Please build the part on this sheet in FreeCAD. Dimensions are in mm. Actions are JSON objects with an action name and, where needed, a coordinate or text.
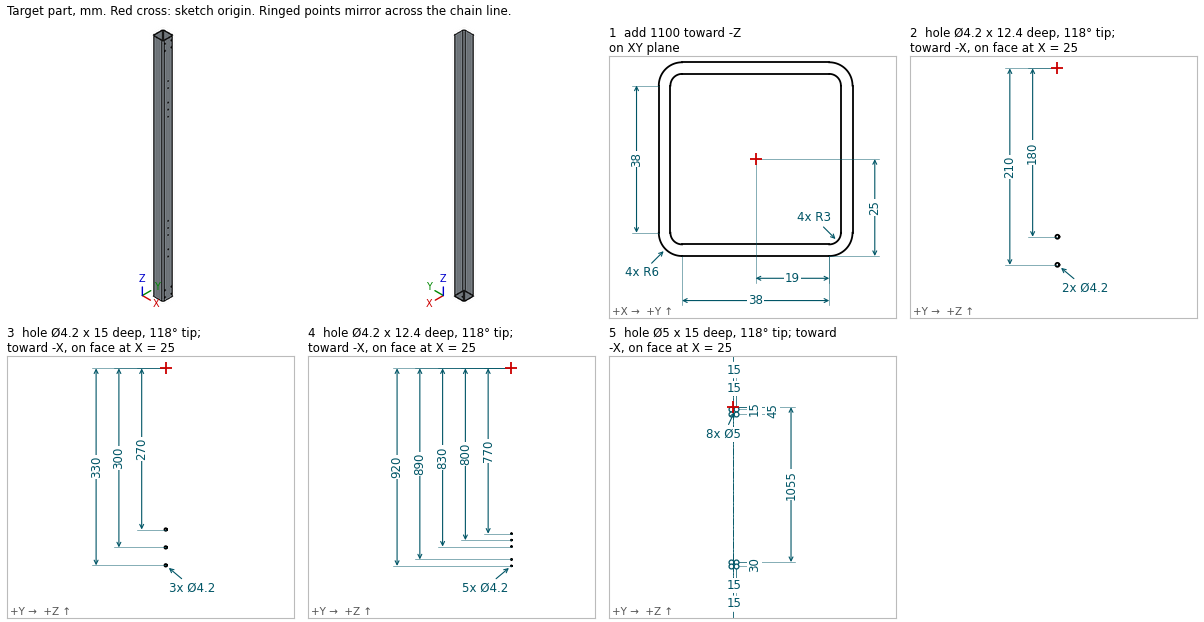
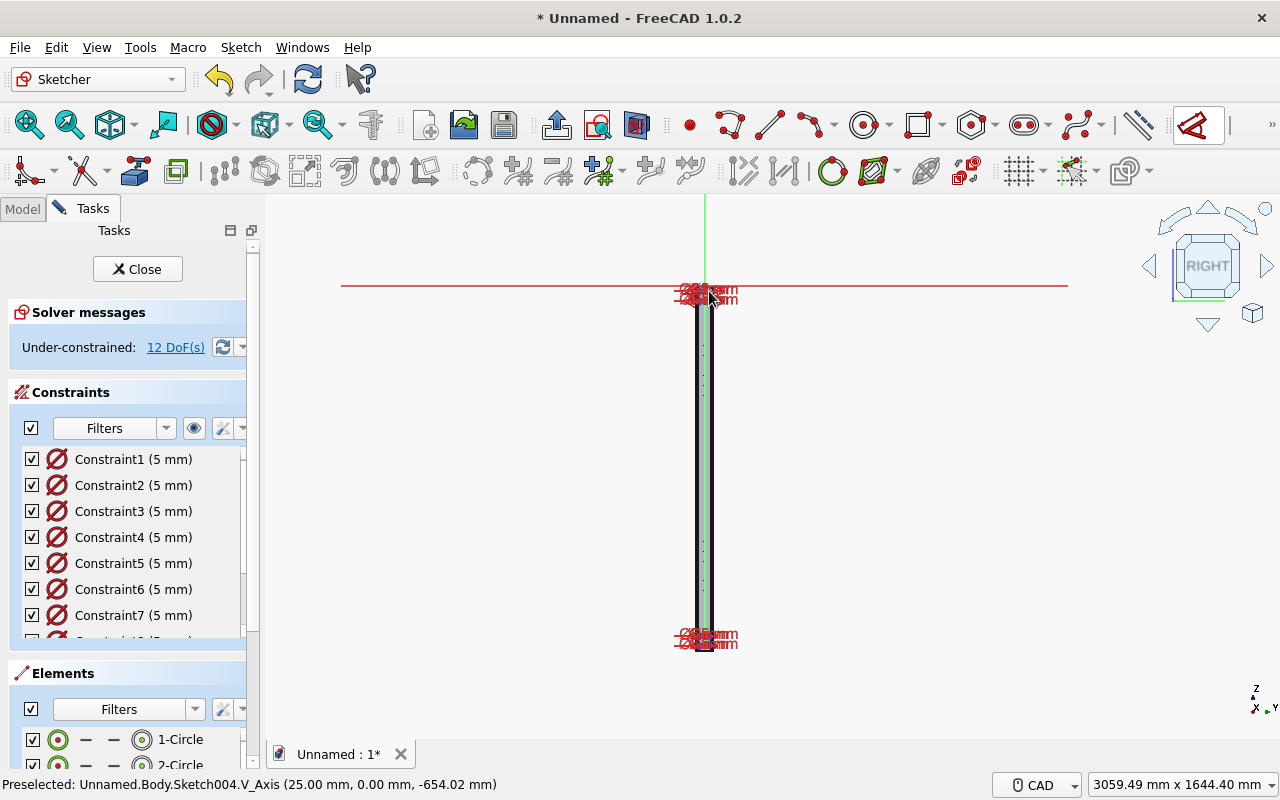
{"action": "scroll", "coordinate": [710, 636], "scroll_direction": "up", "scroll_amount": 2}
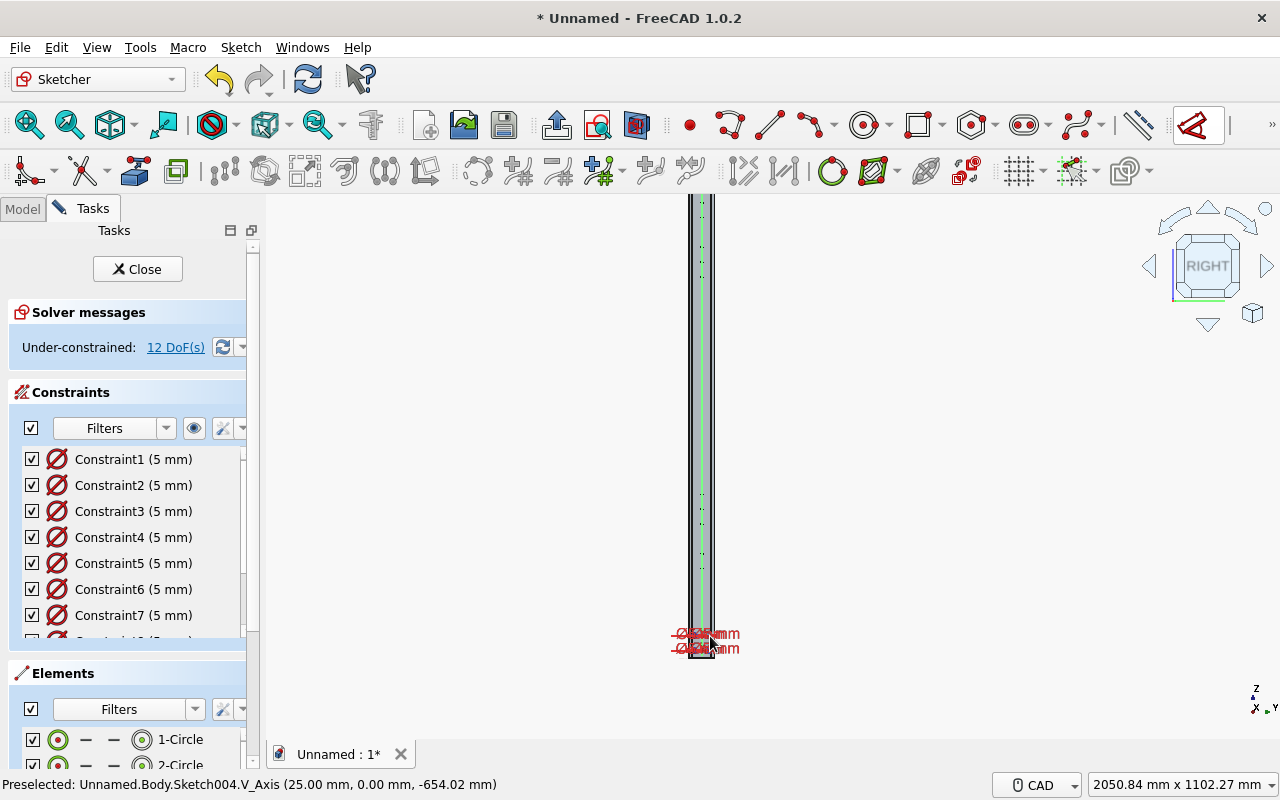
{"action": "left_click", "coordinate": [709, 636]}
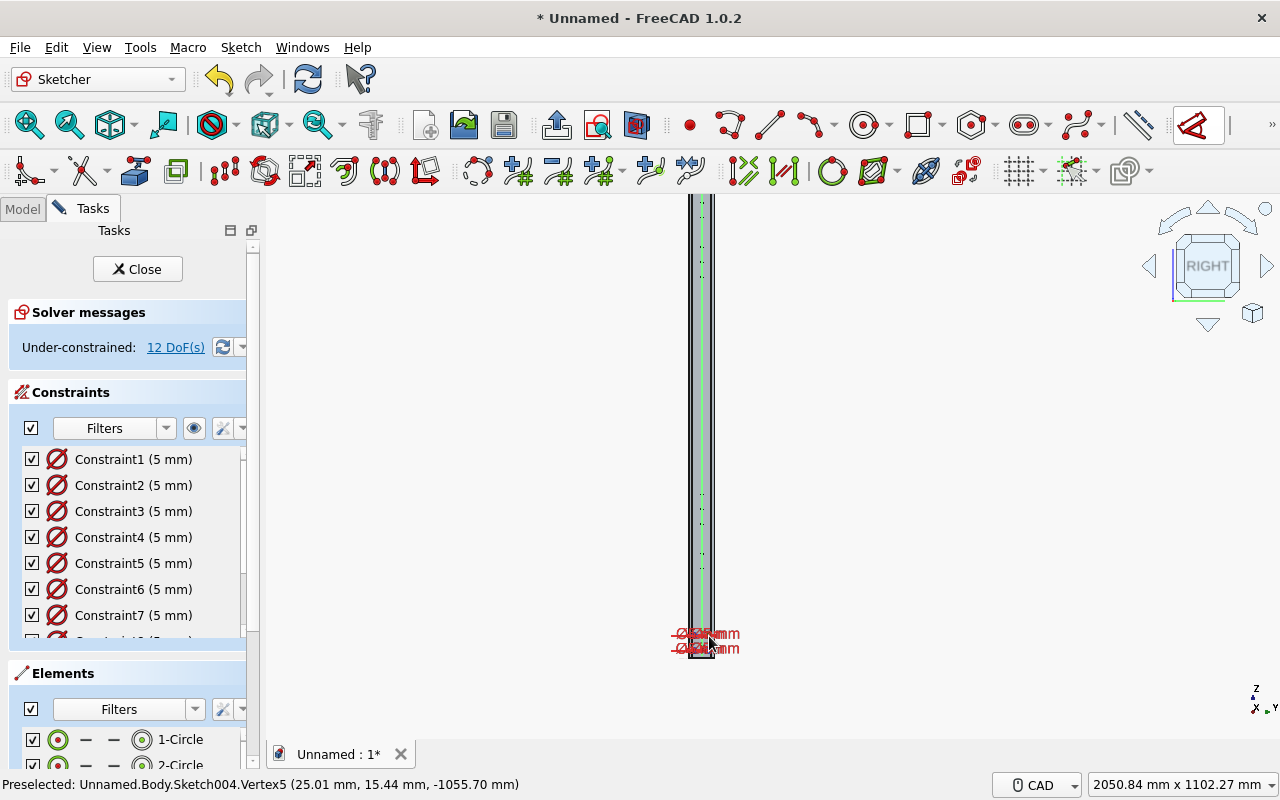
{"action": "left_click", "coordinate": [695, 636]}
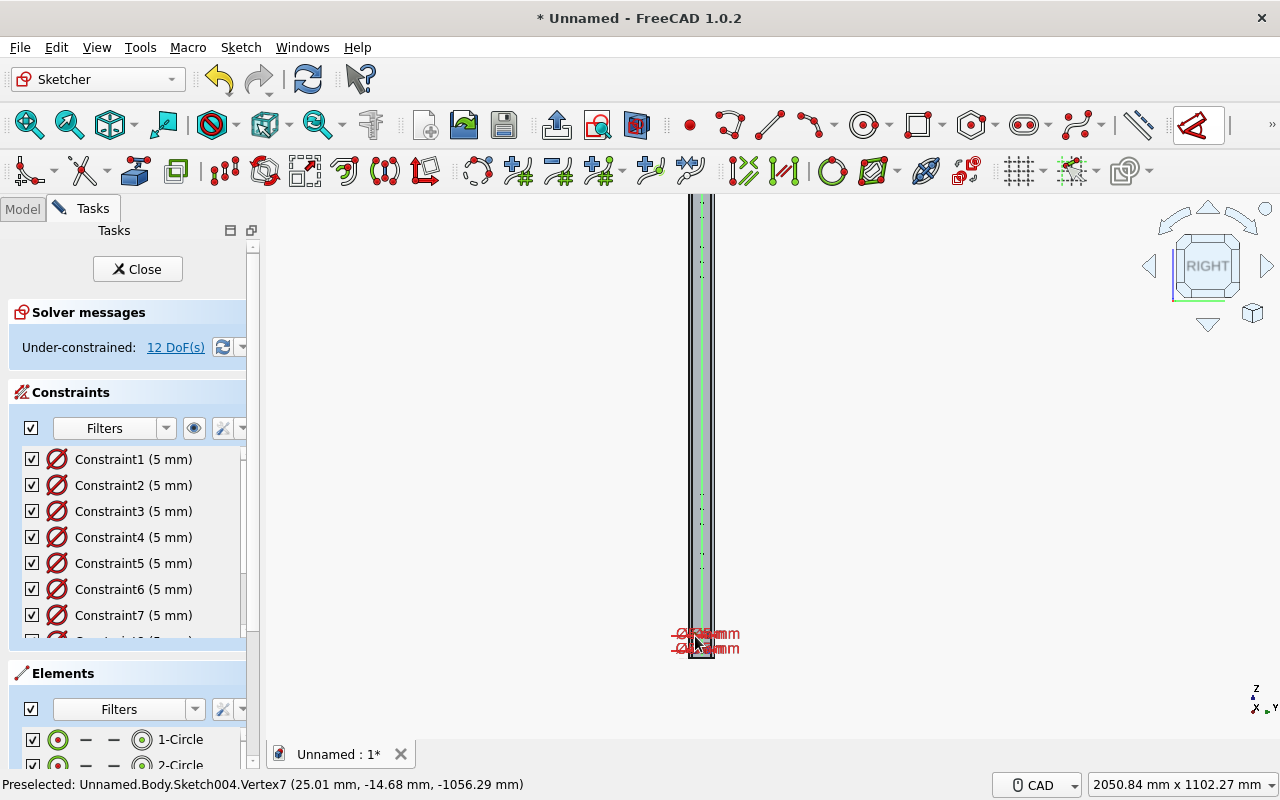
{"action": "left_click", "coordinate": [702, 571]}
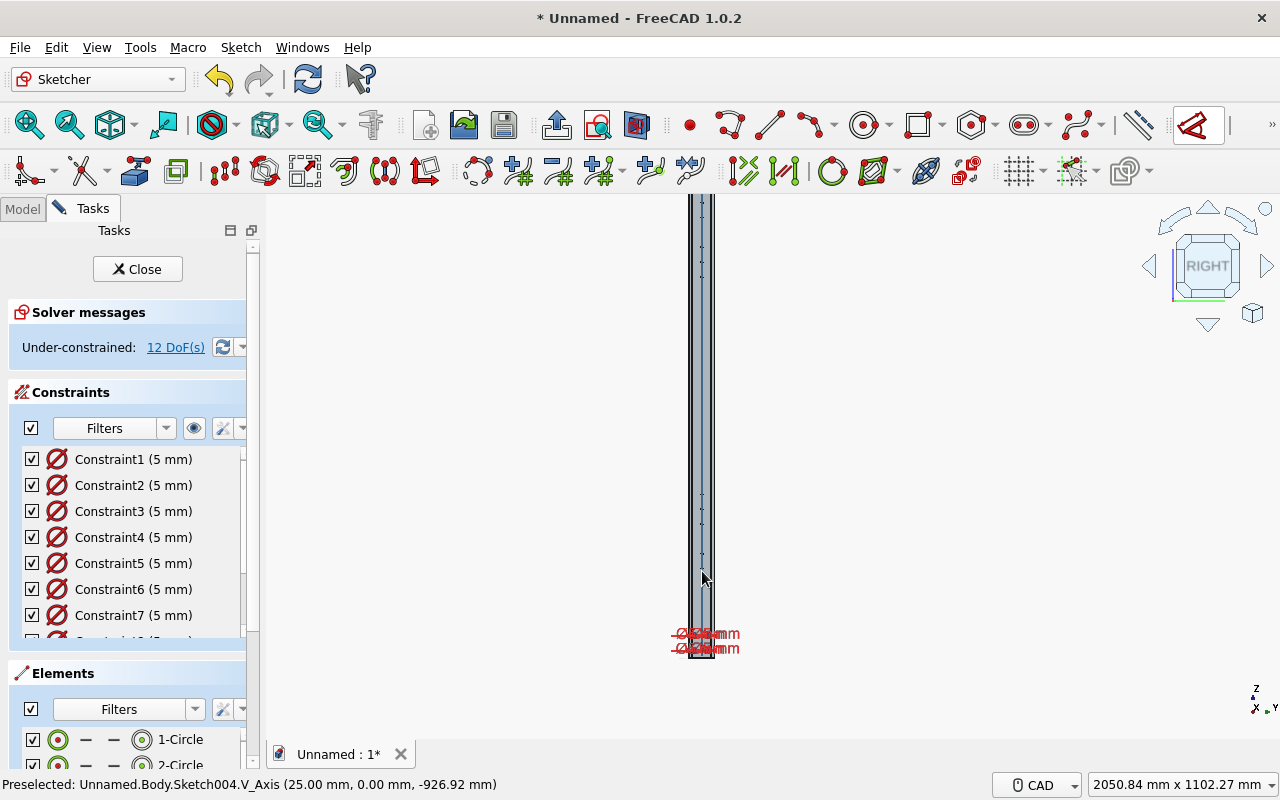
{"action": "key", "text": "s"}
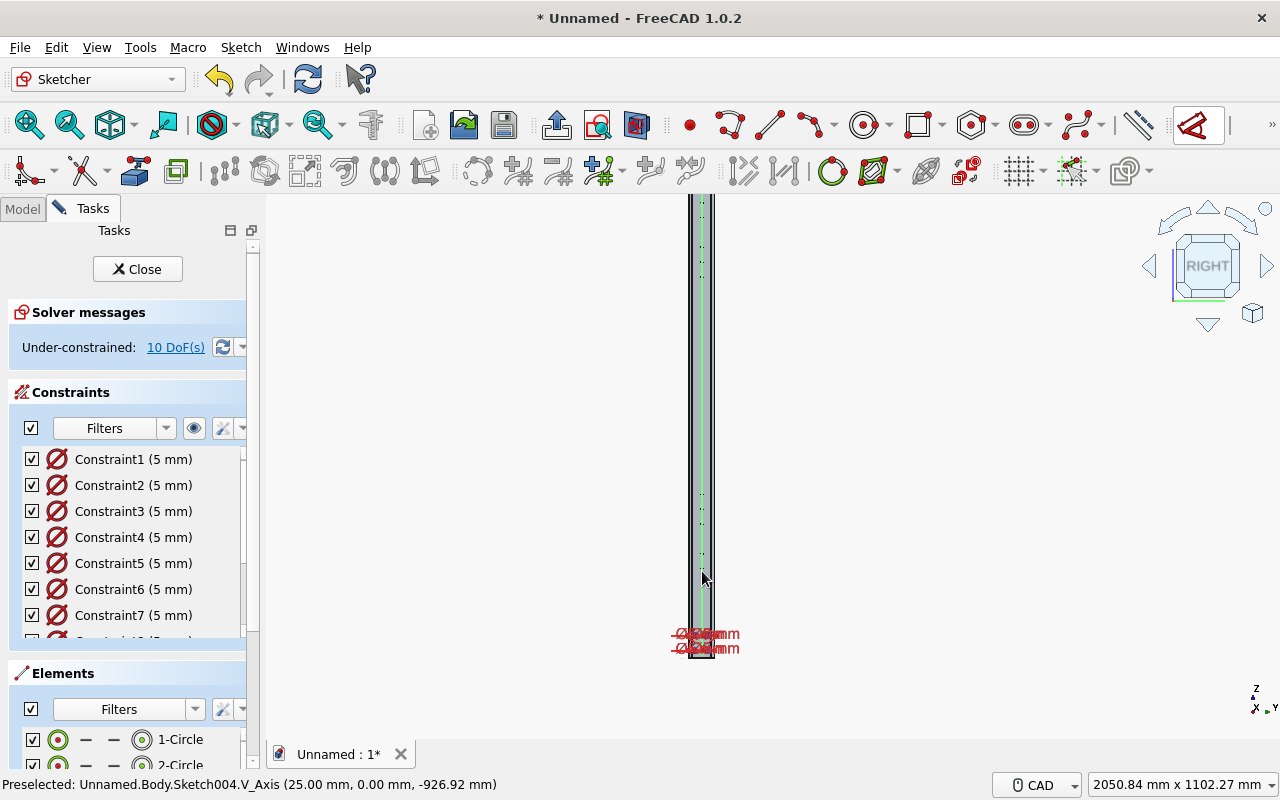
{"action": "left_click", "coordinate": [709, 650]}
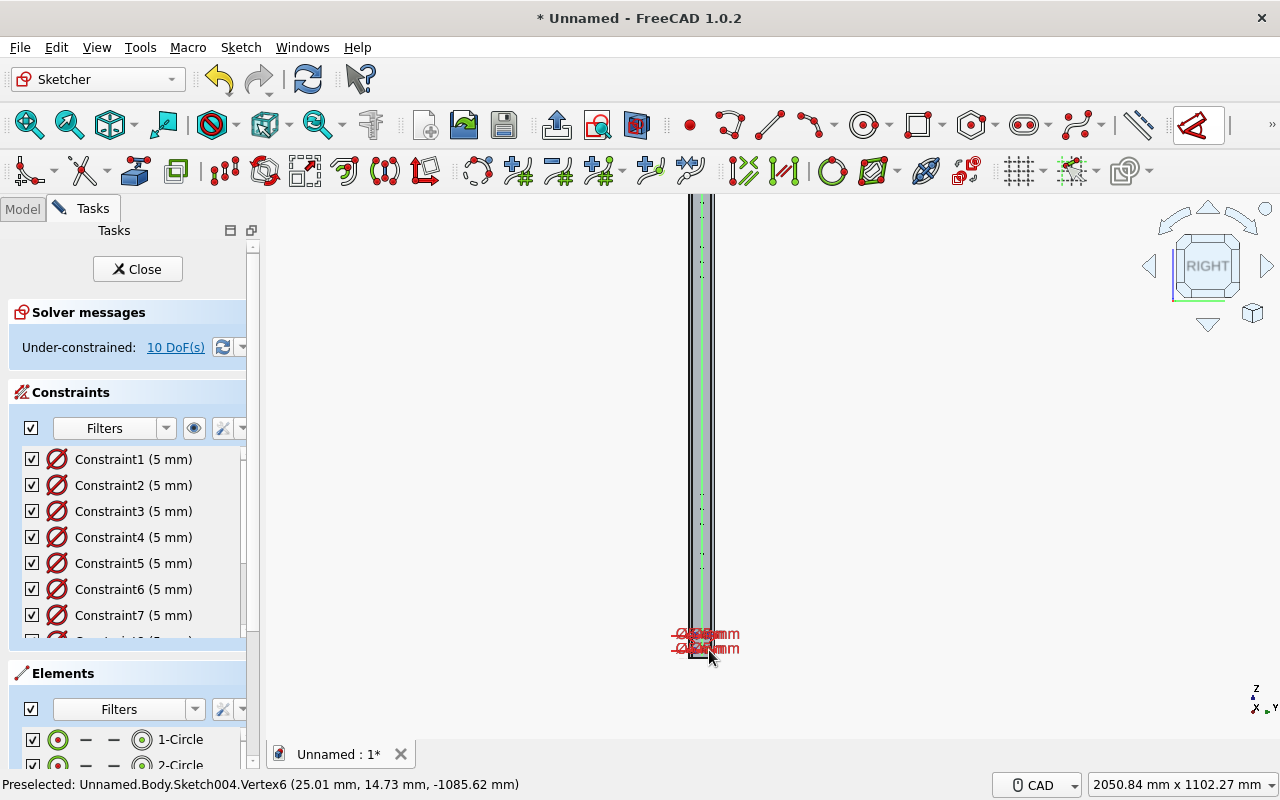
{"action": "left_click", "coordinate": [694, 651]}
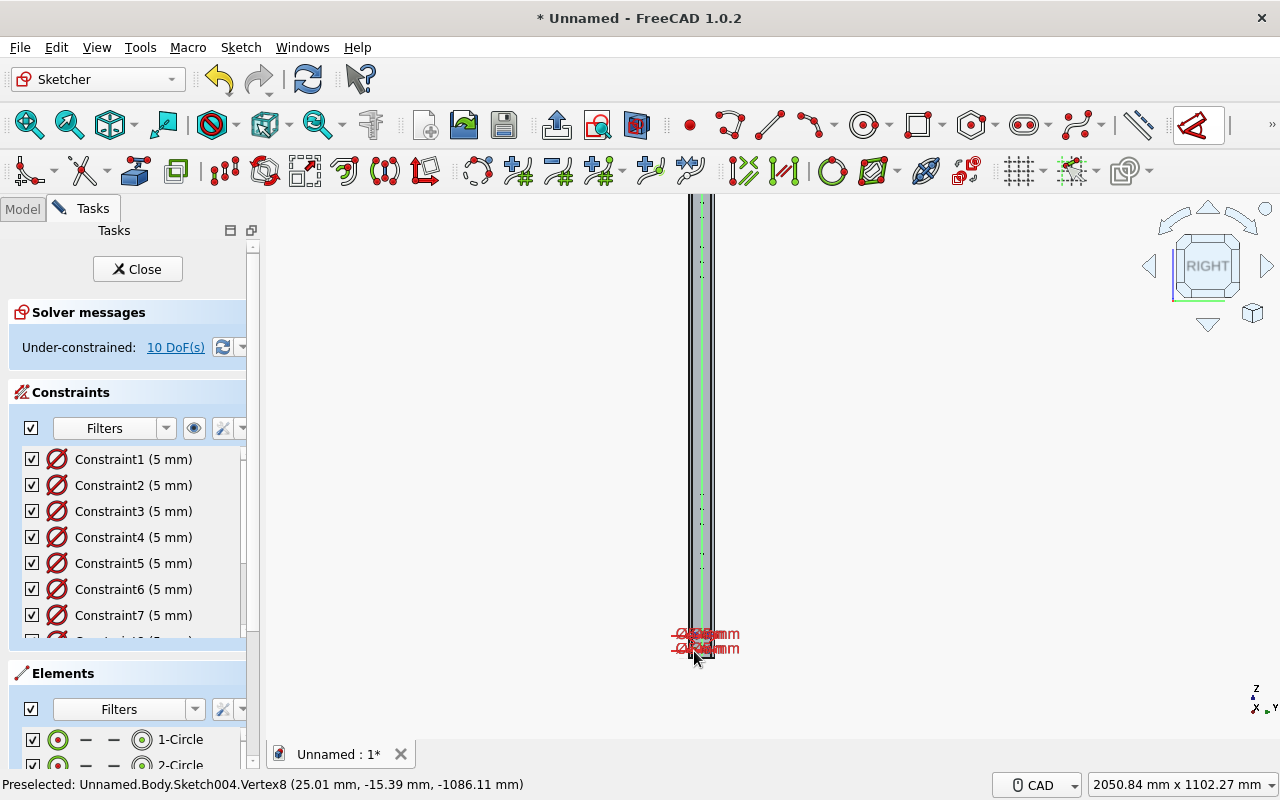
{"action": "left_click", "coordinate": [702, 571]}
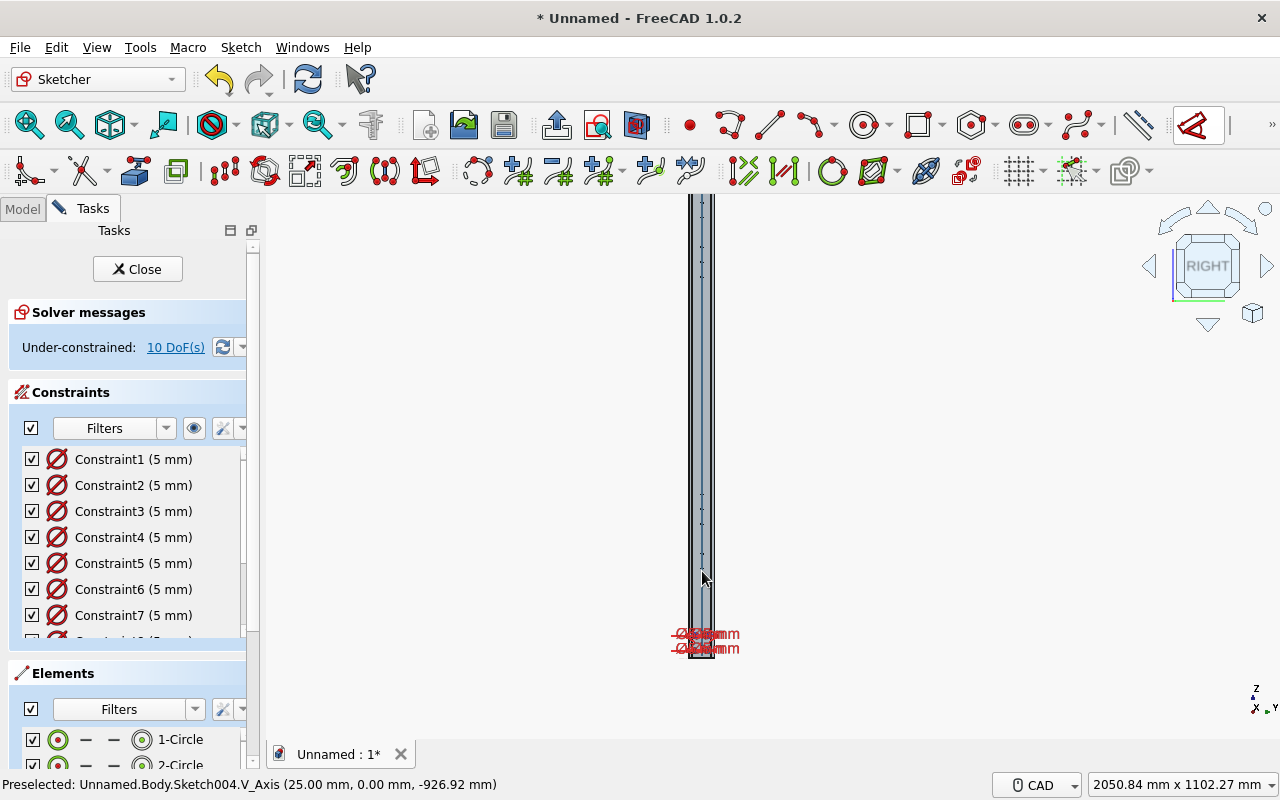
{"action": "key", "text": "s"}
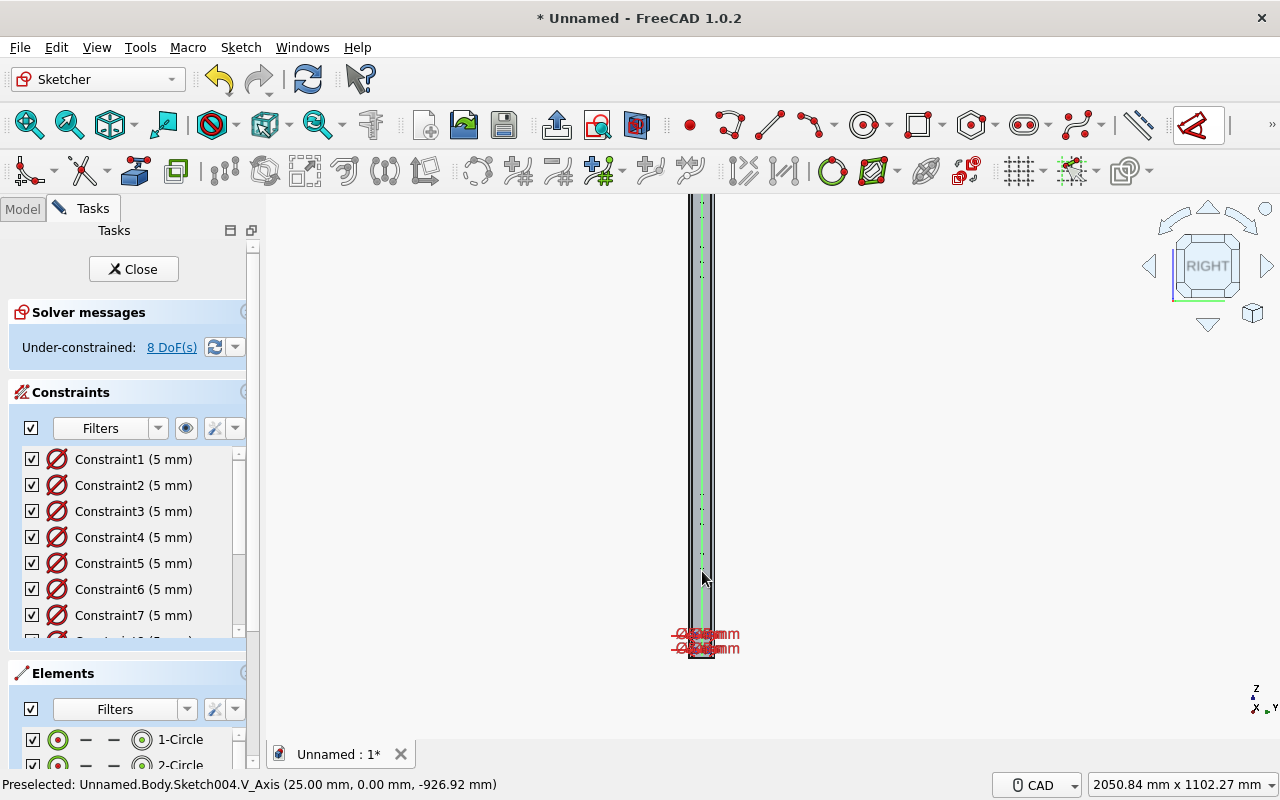
{"action": "scroll", "coordinate": [710, 637], "scroll_direction": "down", "scroll_amount": 2}